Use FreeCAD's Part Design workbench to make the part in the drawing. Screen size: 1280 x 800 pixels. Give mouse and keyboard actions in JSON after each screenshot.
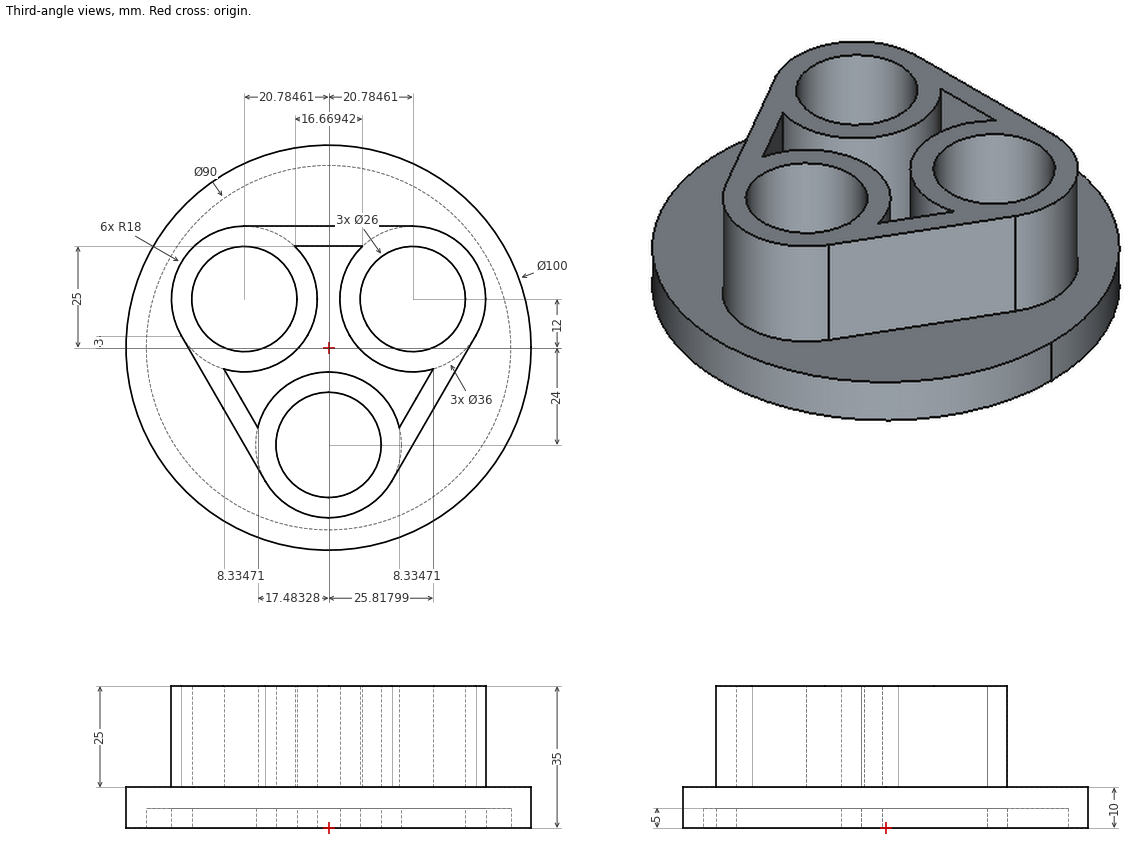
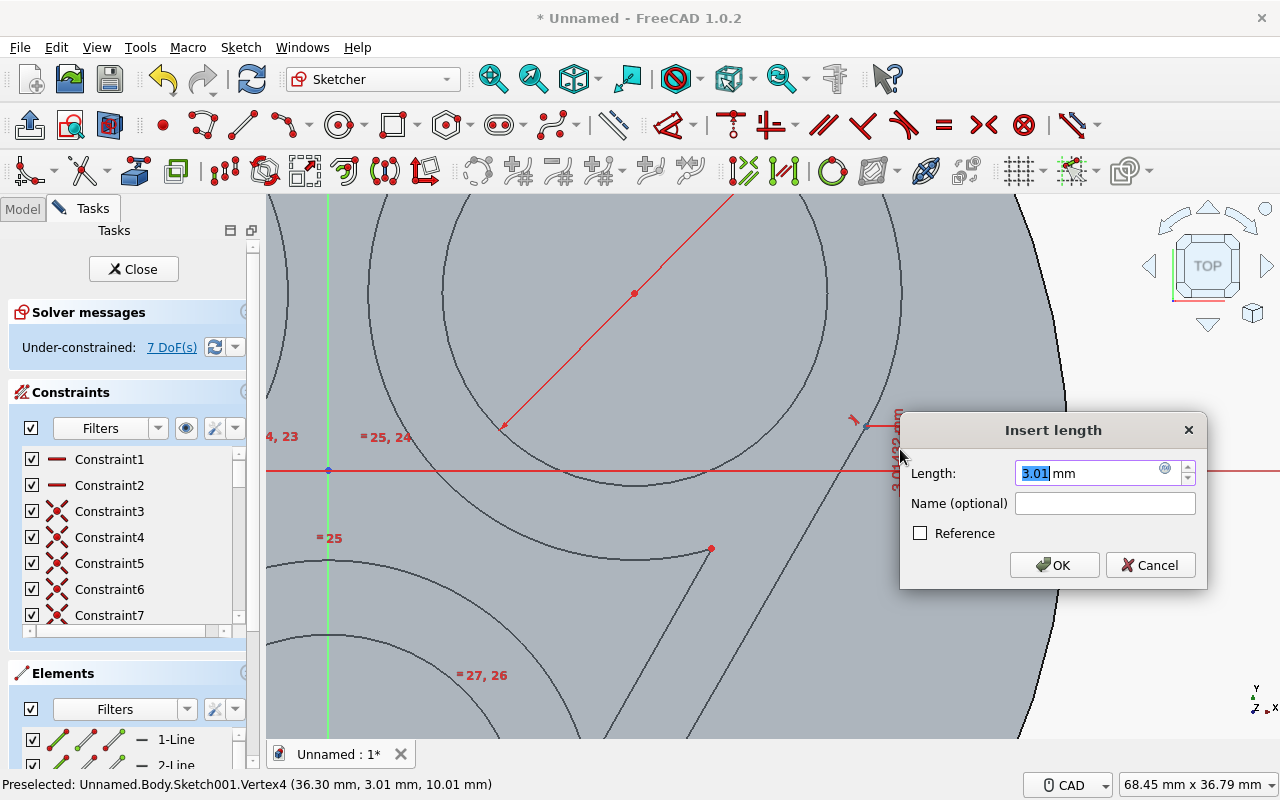
{"action": "type", "text": "3"}
{"action": "key", "text": "Return"}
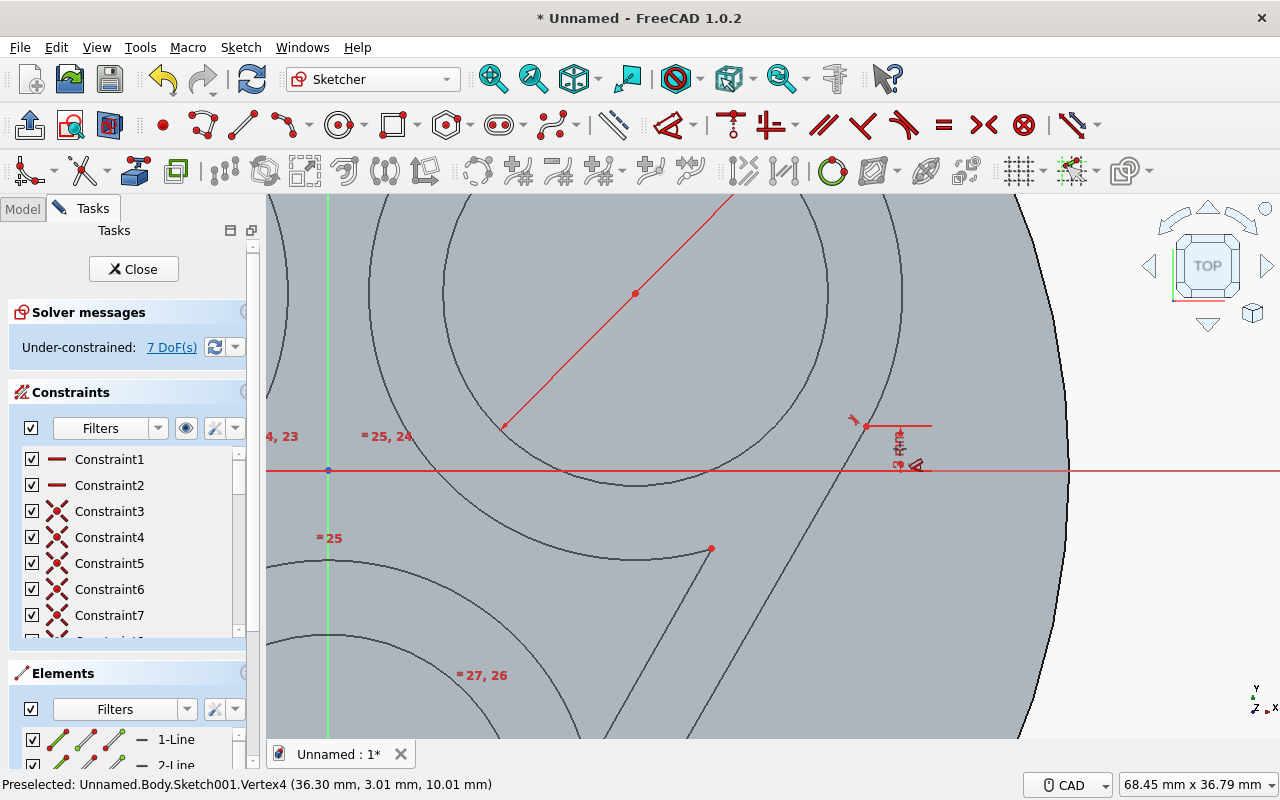
{"action": "scroll", "coordinate": [867, 426], "scroll_direction": "down", "scroll_amount": 6}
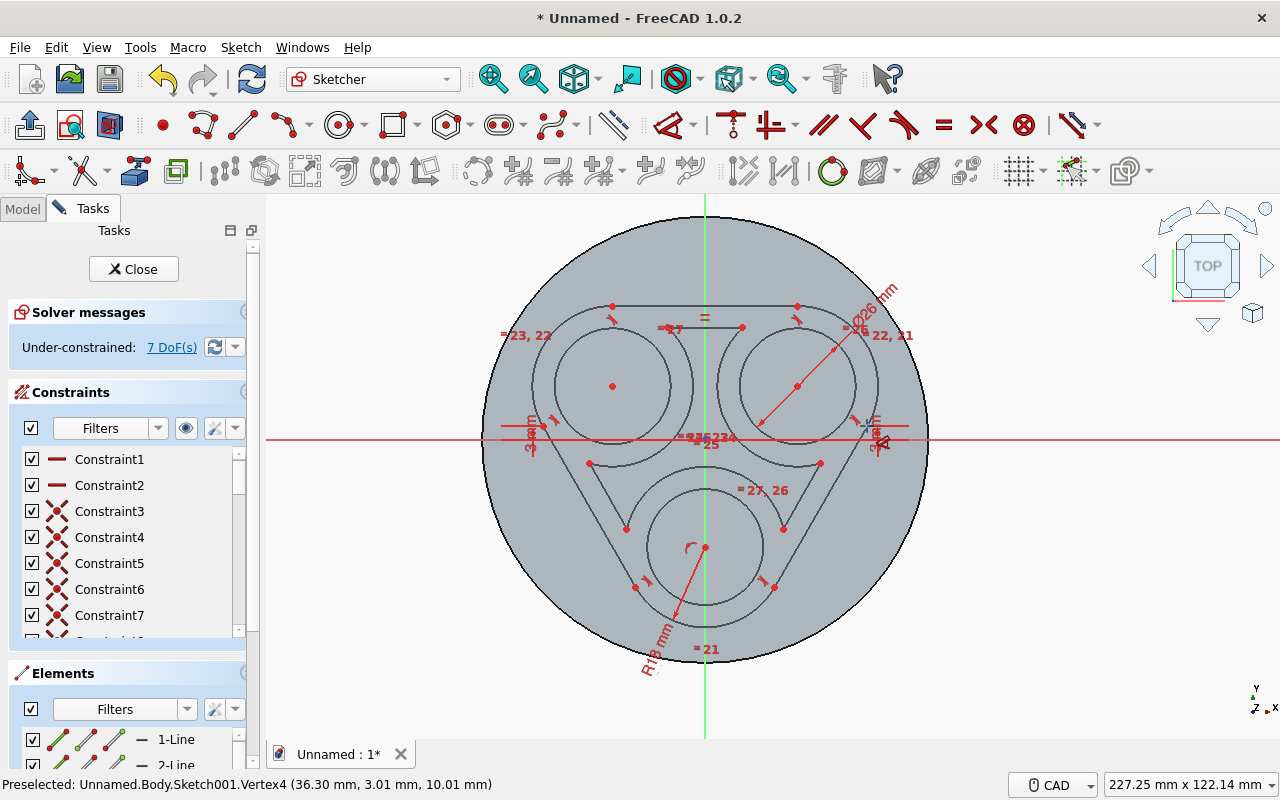
{"action": "left_click", "coordinate": [705, 547]}
{"action": "left_click", "coordinate": [671, 518]}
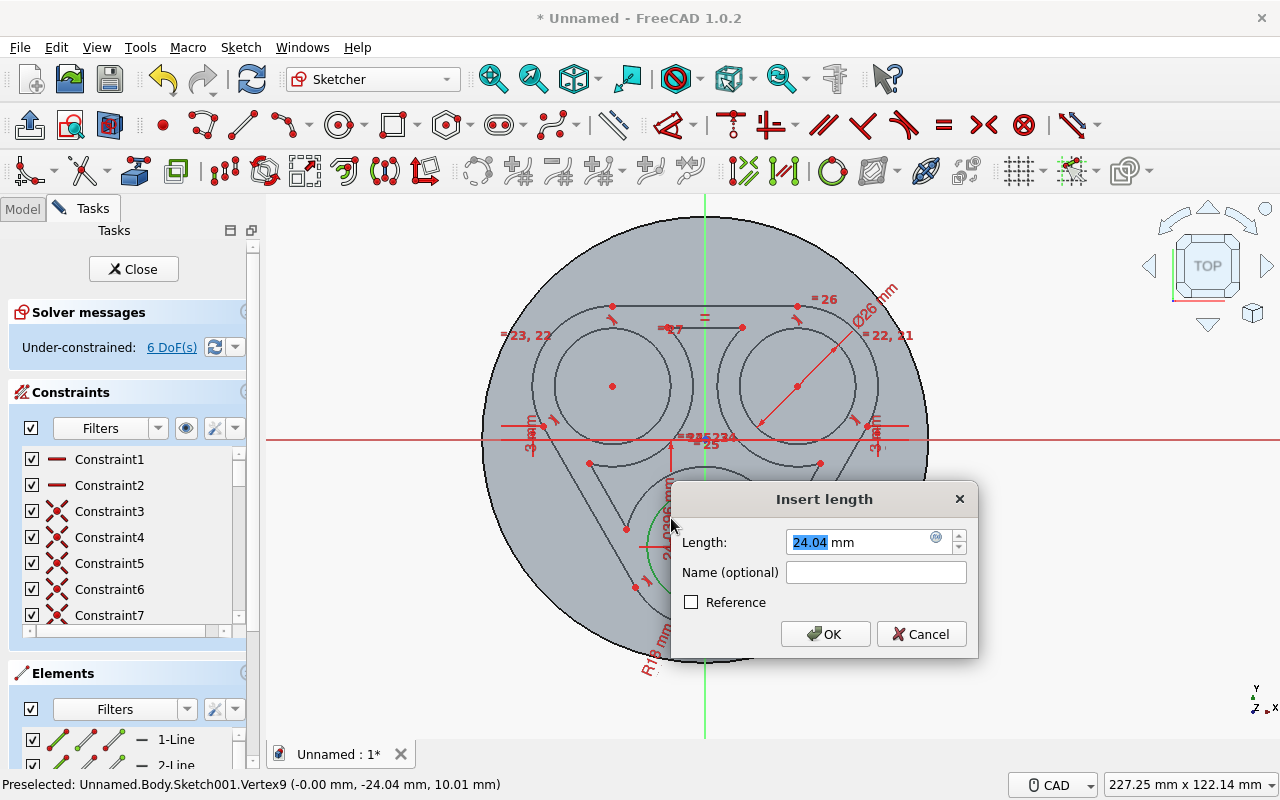
{"action": "type", "text": "24"}
{"action": "key", "text": "Return"}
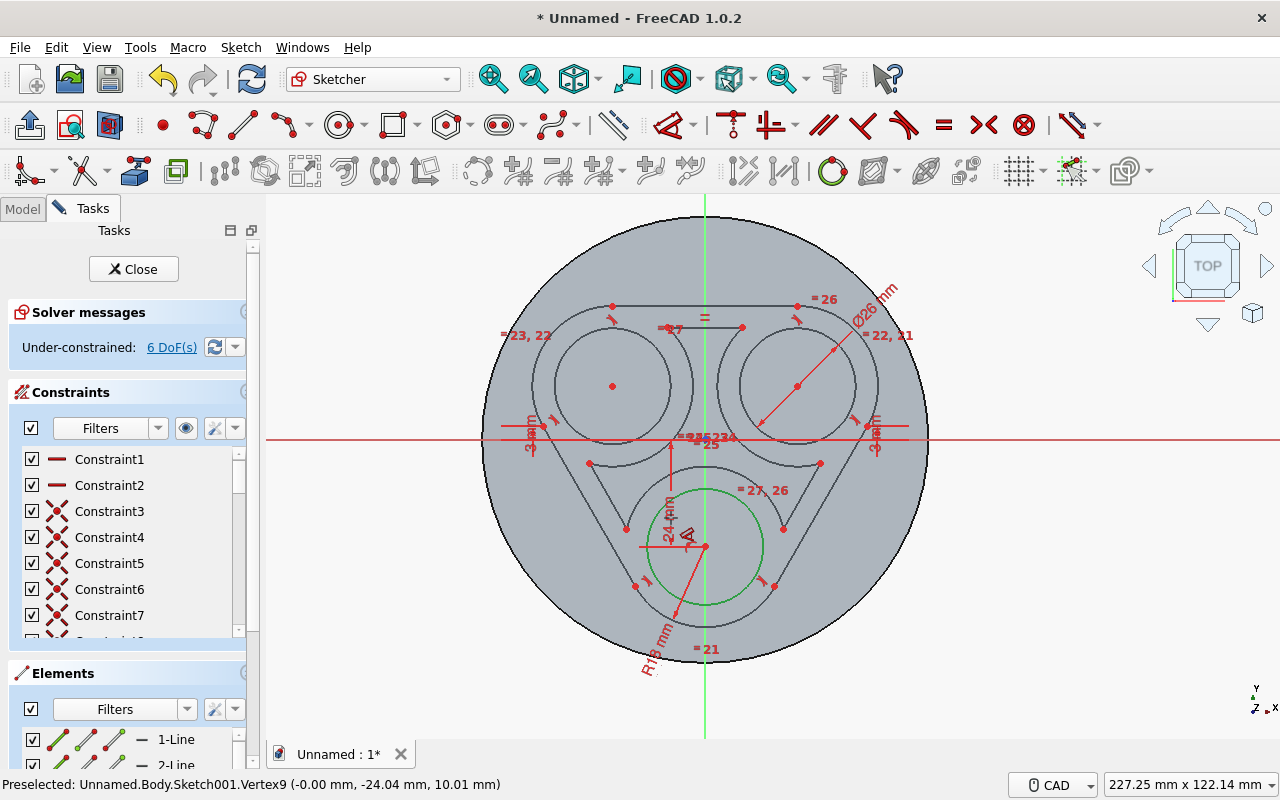
{"action": "left_click", "coordinate": [668, 328]}
{"action": "left_click", "coordinate": [634, 384]}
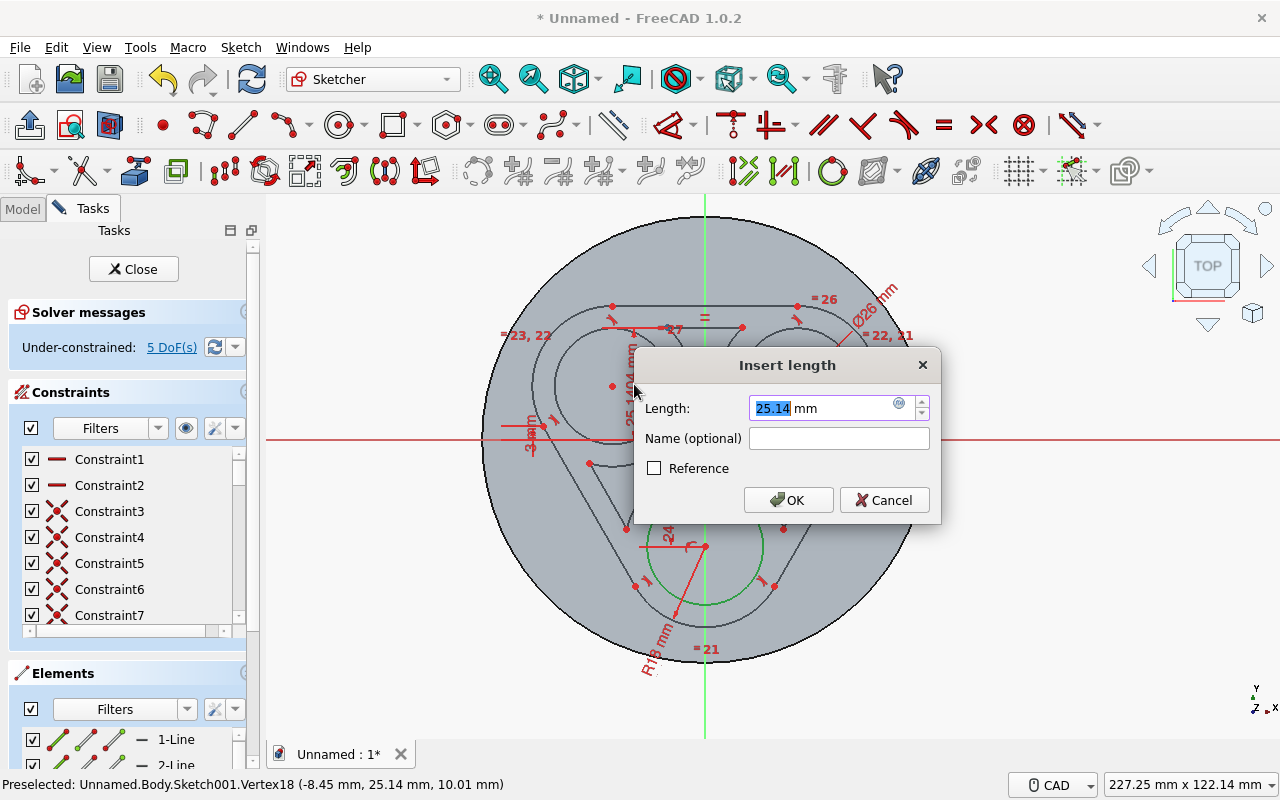
{"action": "type", "text": "25"}
{"action": "key", "text": "Return"}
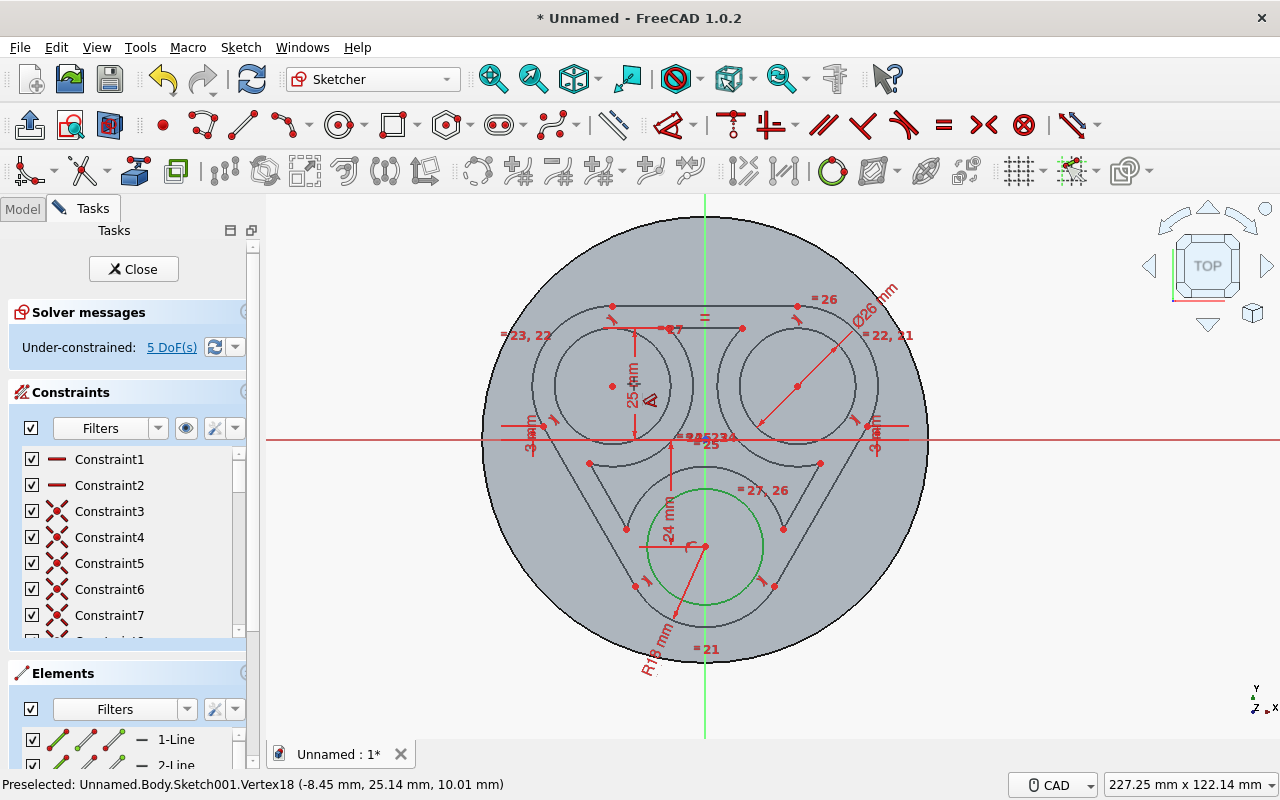
{"action": "left_click", "coordinate": [690, 328]}
{"action": "left_click", "coordinate": [688, 270]}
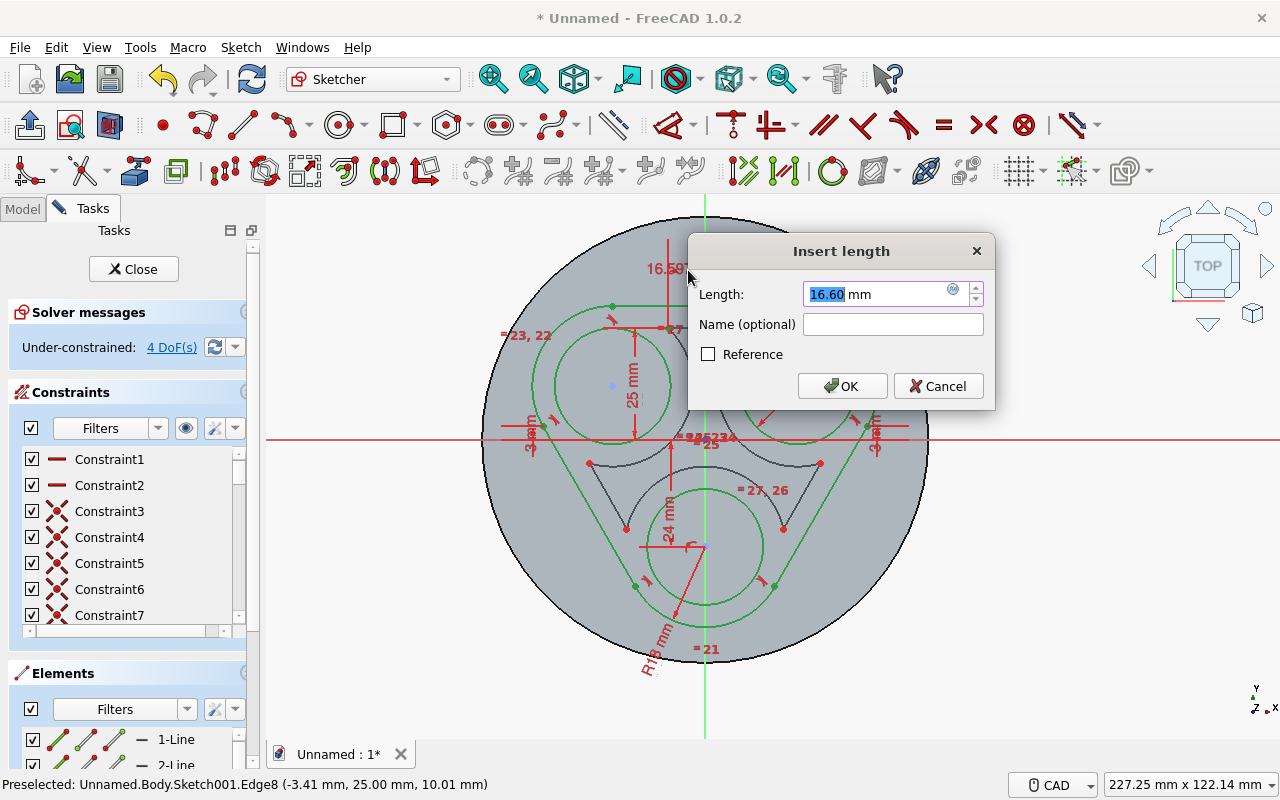
{"action": "type", "text": "16.66942"}
{"action": "key", "text": "Return"}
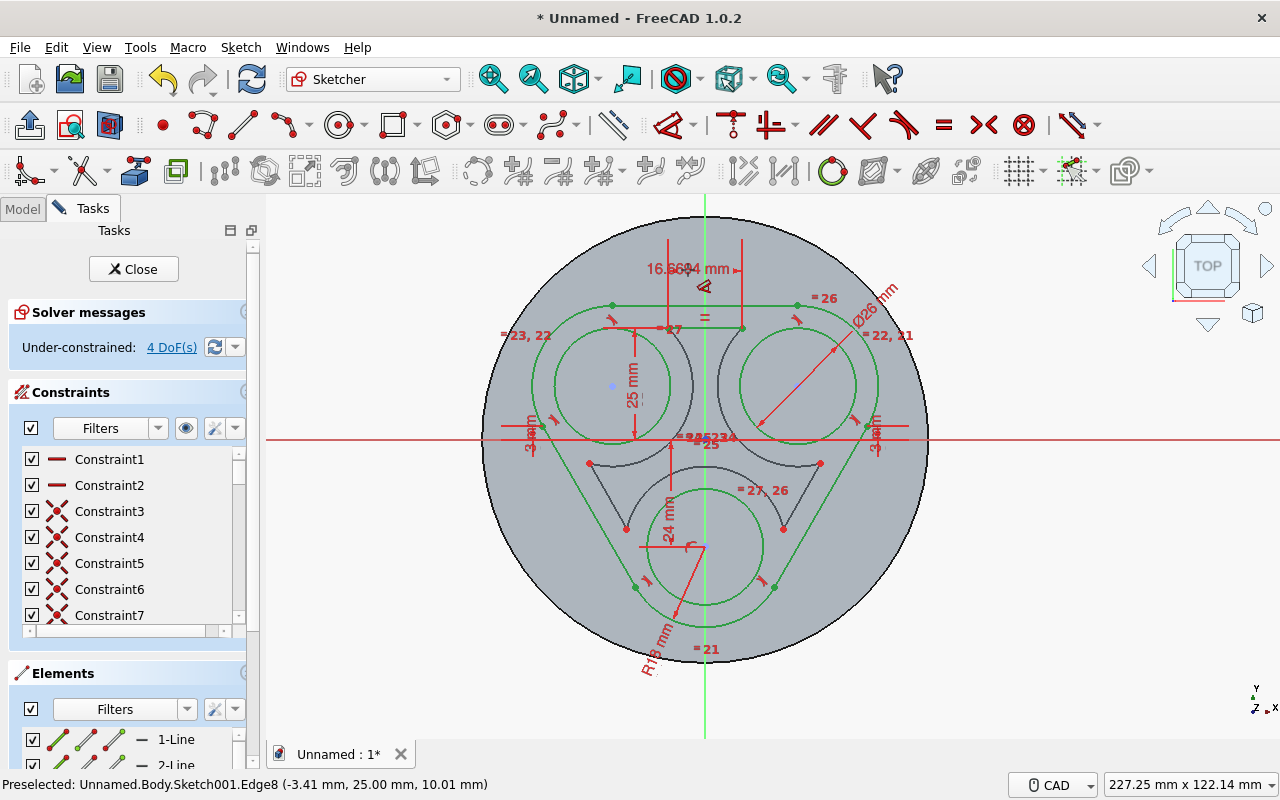
{"action": "left_click", "coordinate": [616, 509]}
{"action": "left_click", "coordinate": [600, 563]}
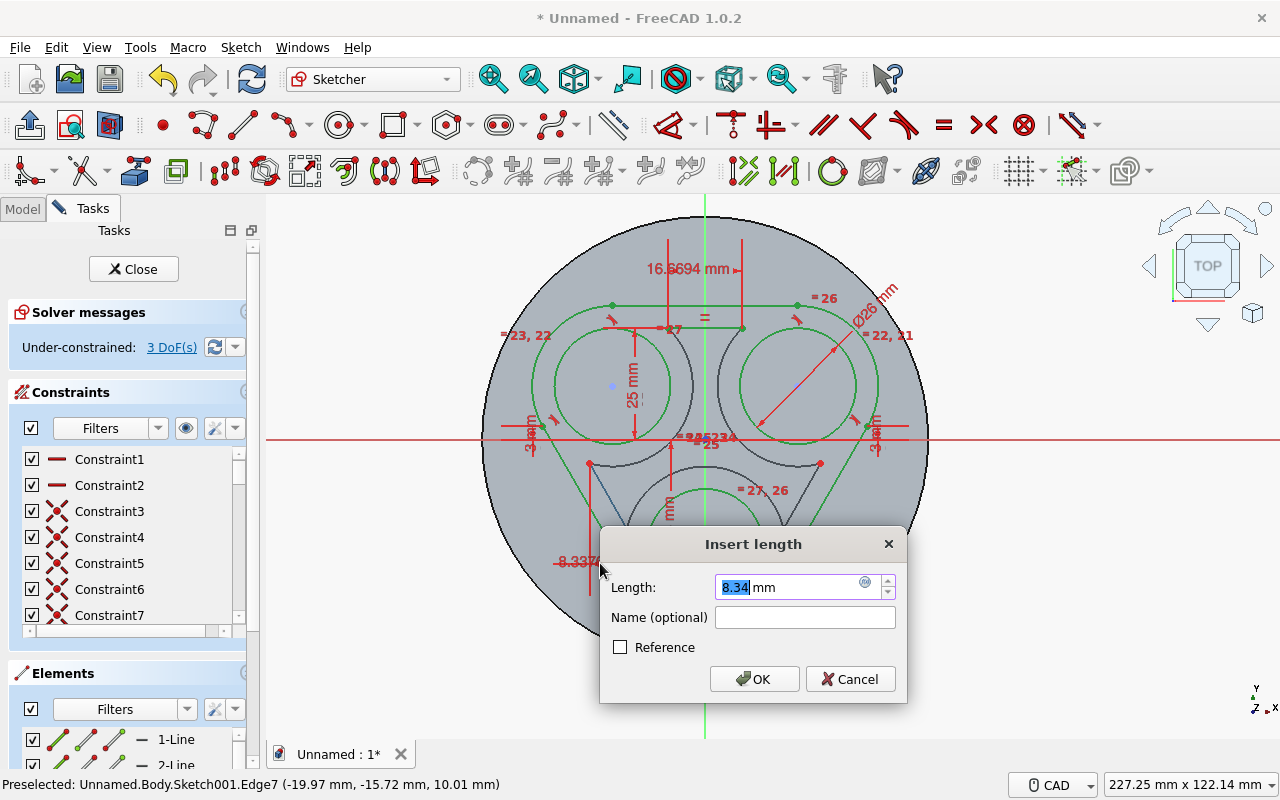
{"action": "type", "text": "8.33471"}
{"action": "key", "text": "Return"}